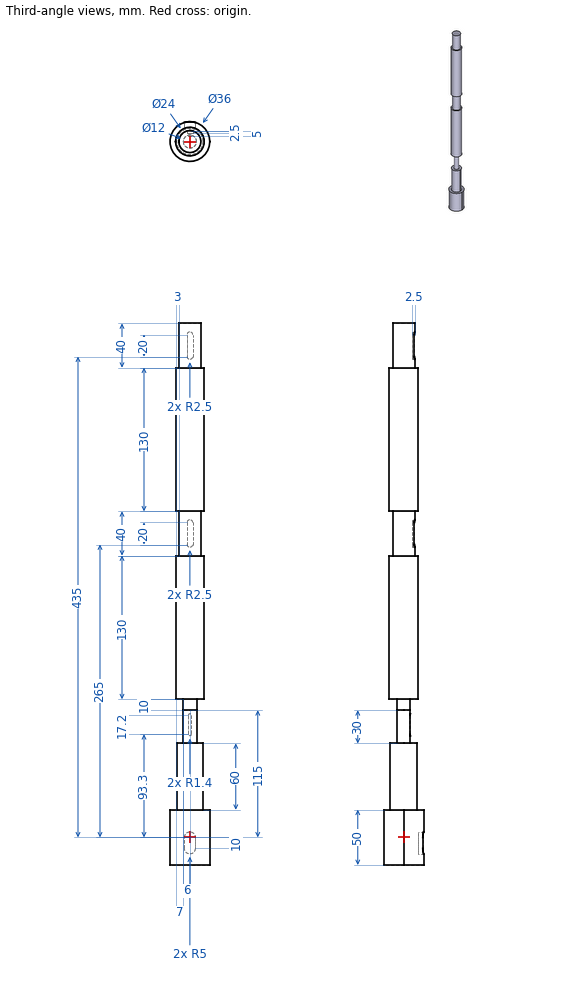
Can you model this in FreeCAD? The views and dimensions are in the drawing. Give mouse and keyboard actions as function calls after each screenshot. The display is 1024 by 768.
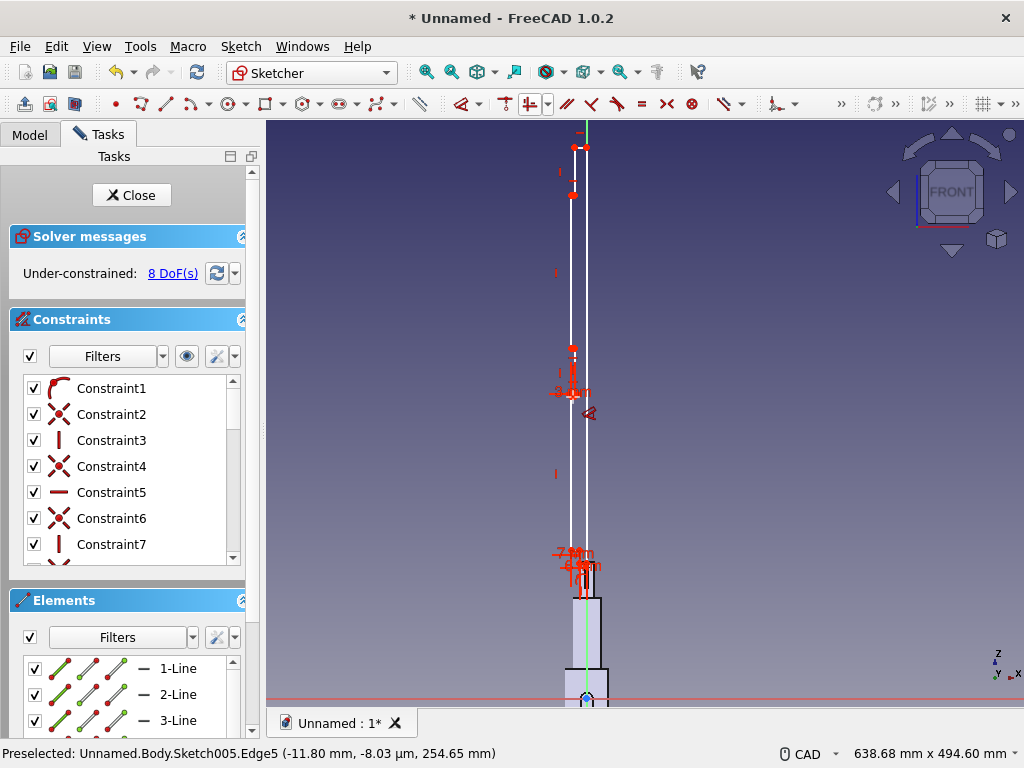
scroll(574, 365, up, 15)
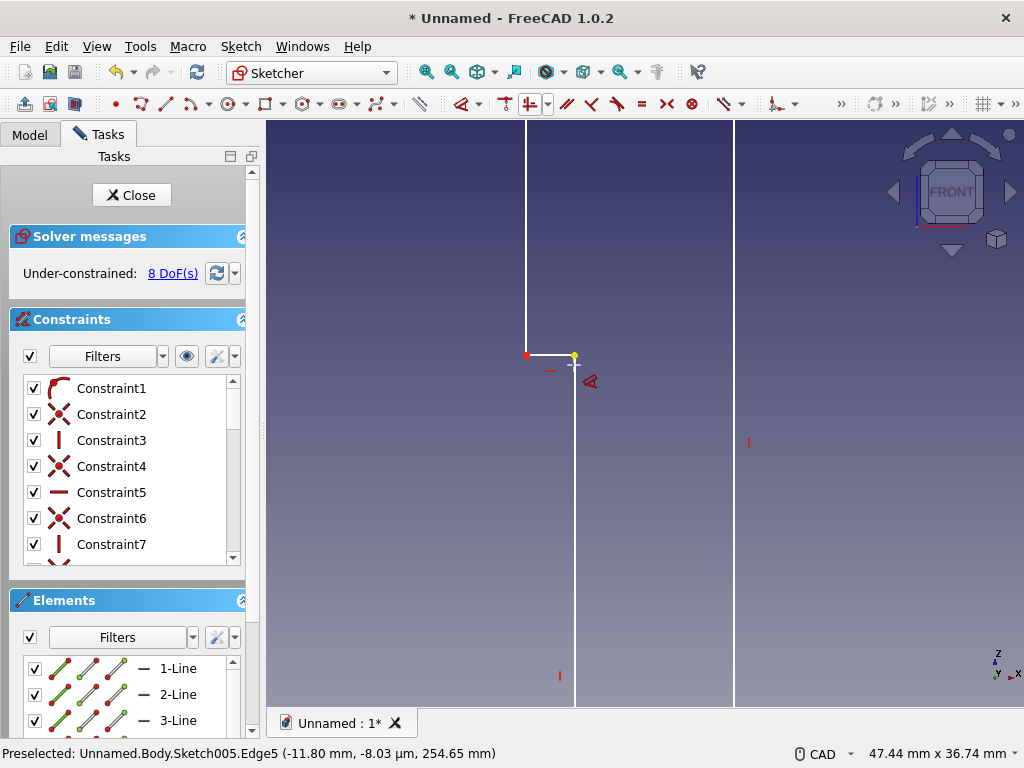
click(560, 355)
click(550, 321)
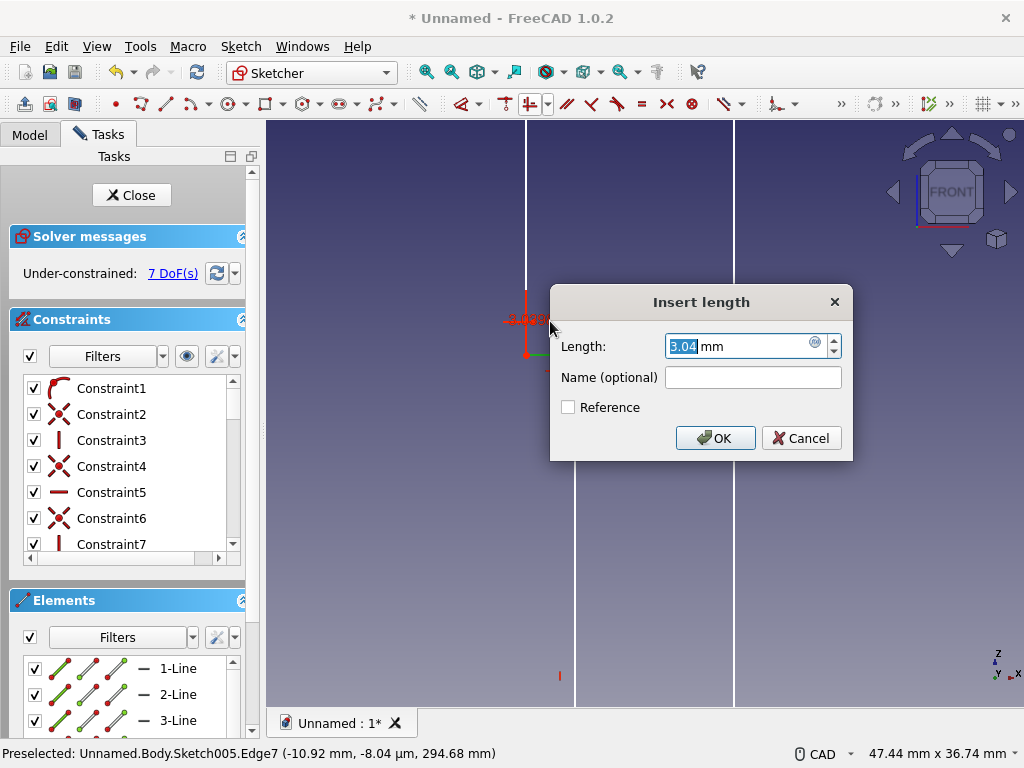
text(3)
key(Return)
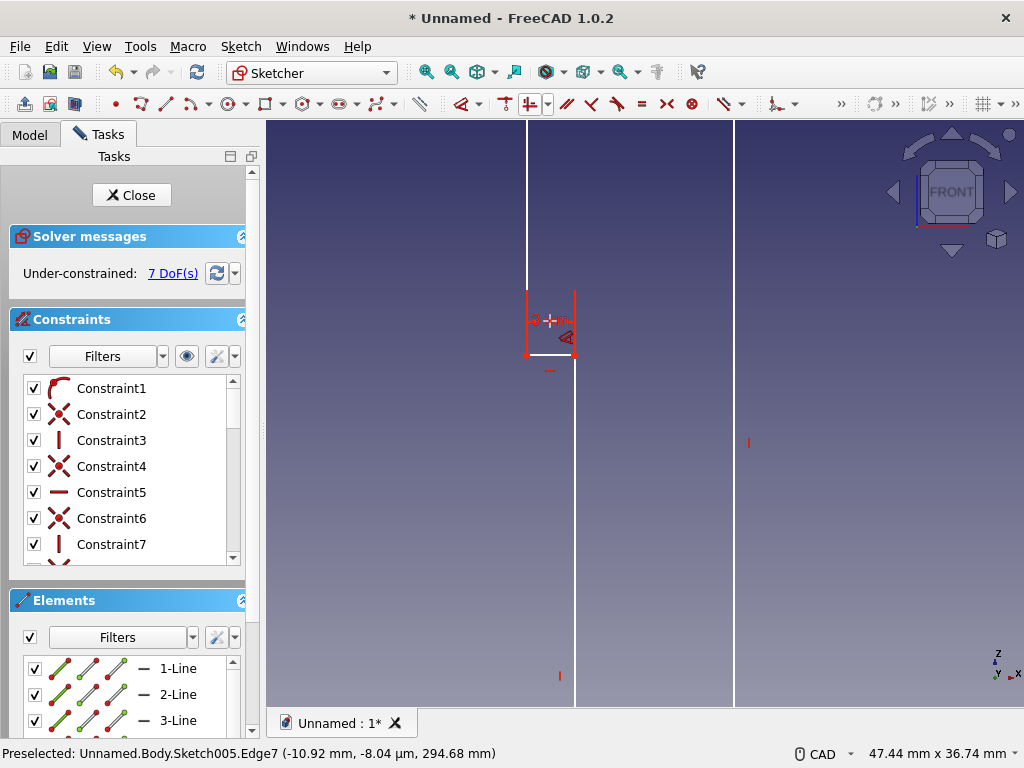
scroll(574, 364, down, 15)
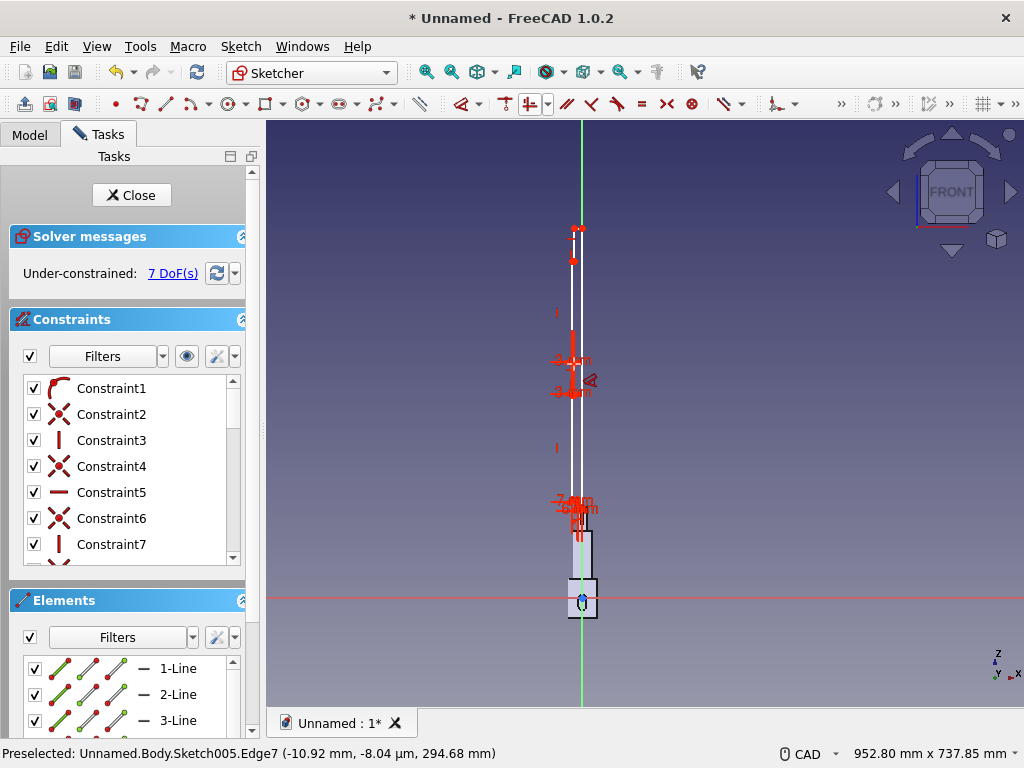
scroll(573, 261, up, 15)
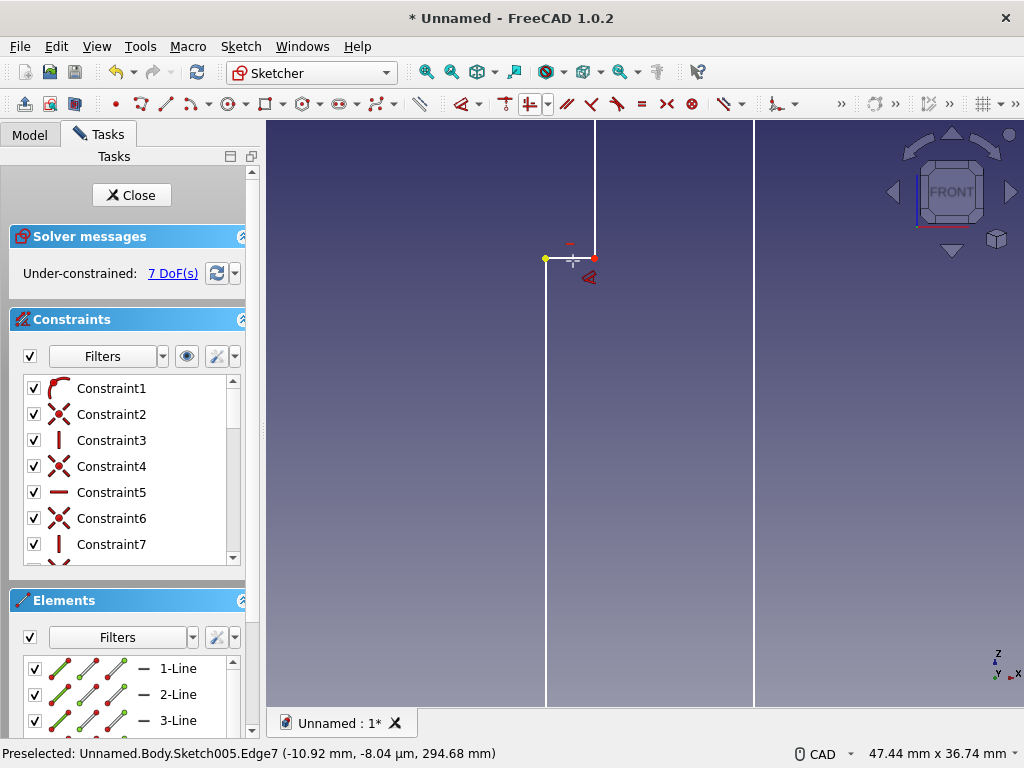
click(561, 258)
click(570, 224)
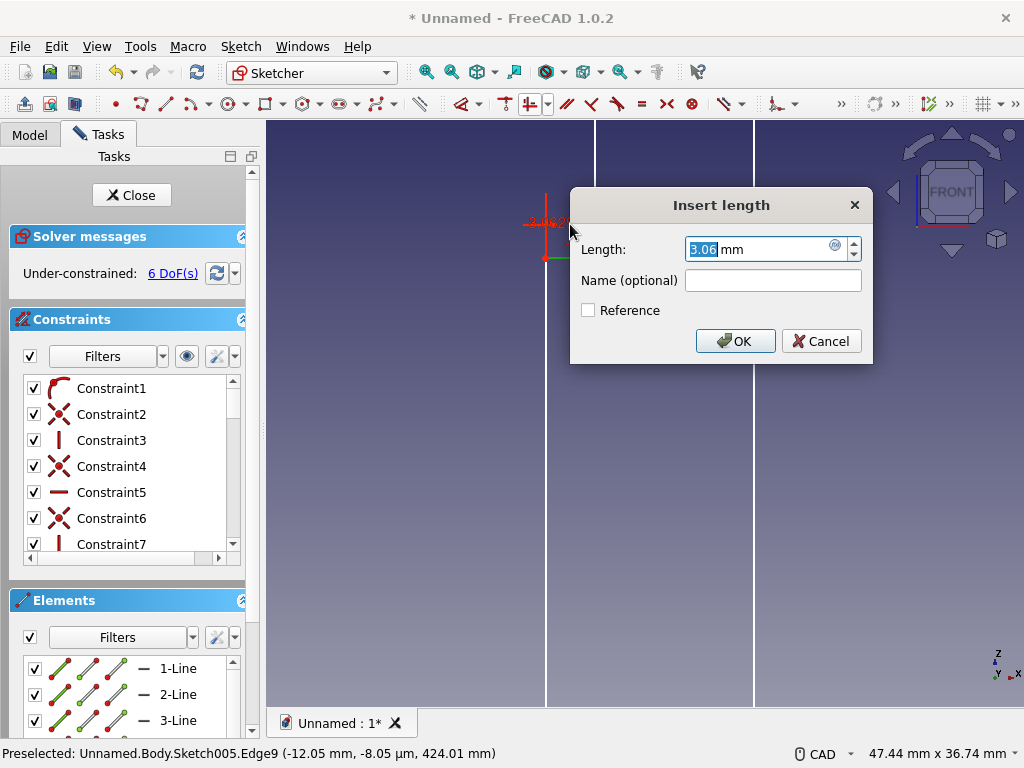
text(3)
key(Return)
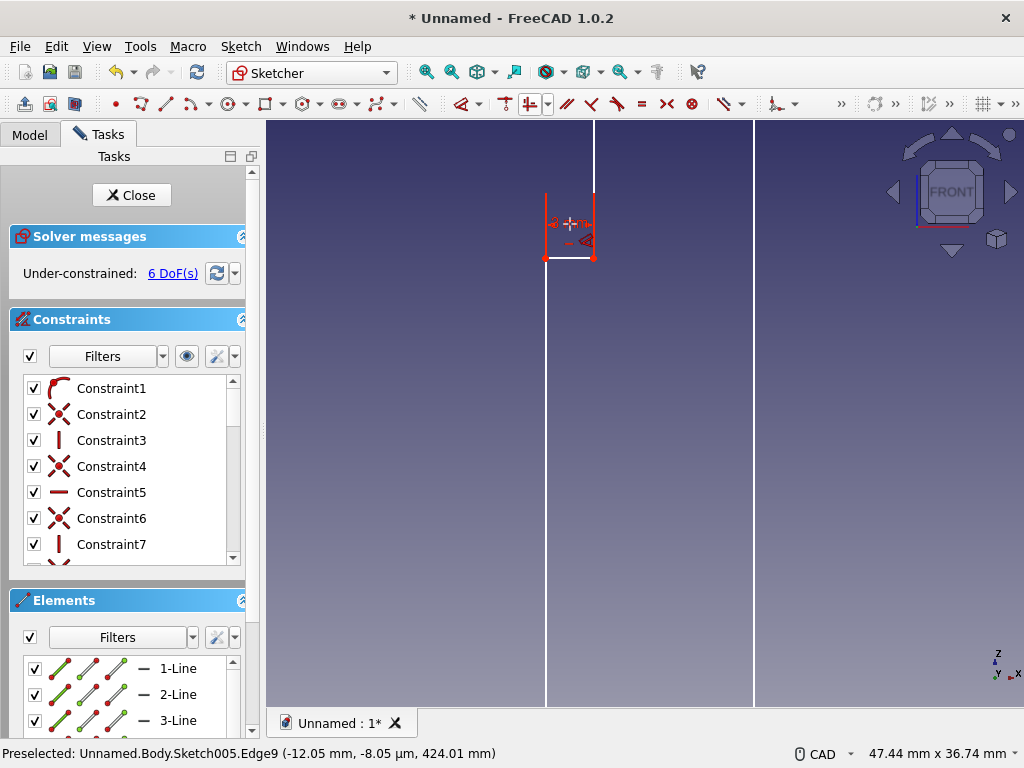
scroll(573, 261, down, 15)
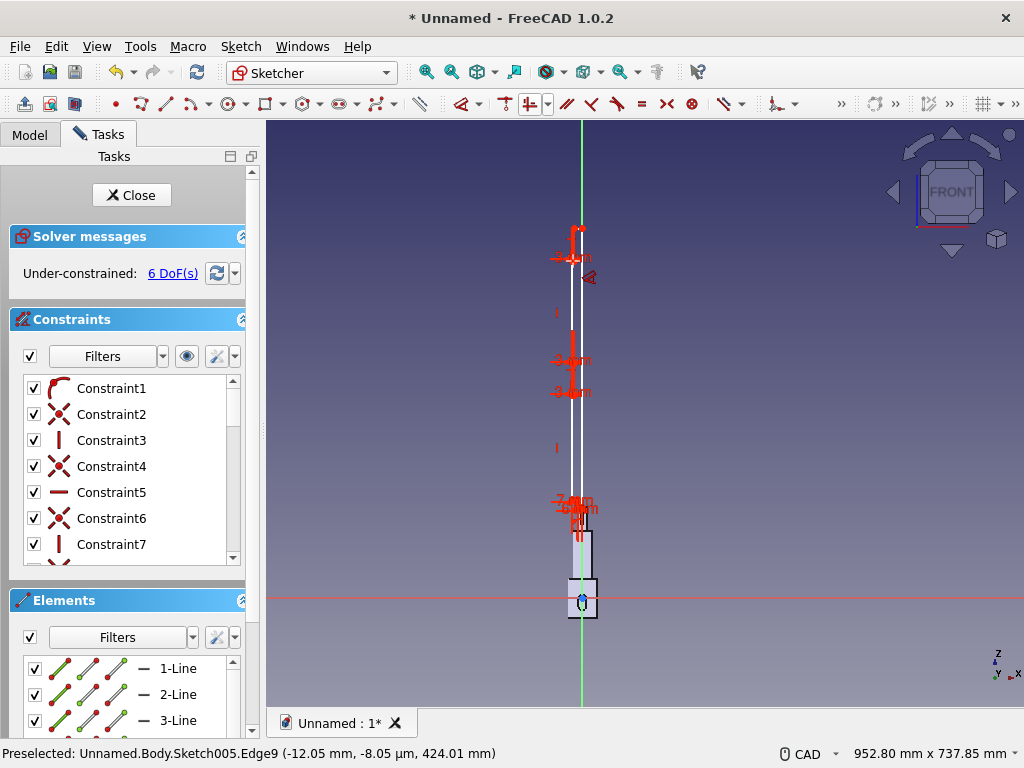
scroll(578, 505, up, 9)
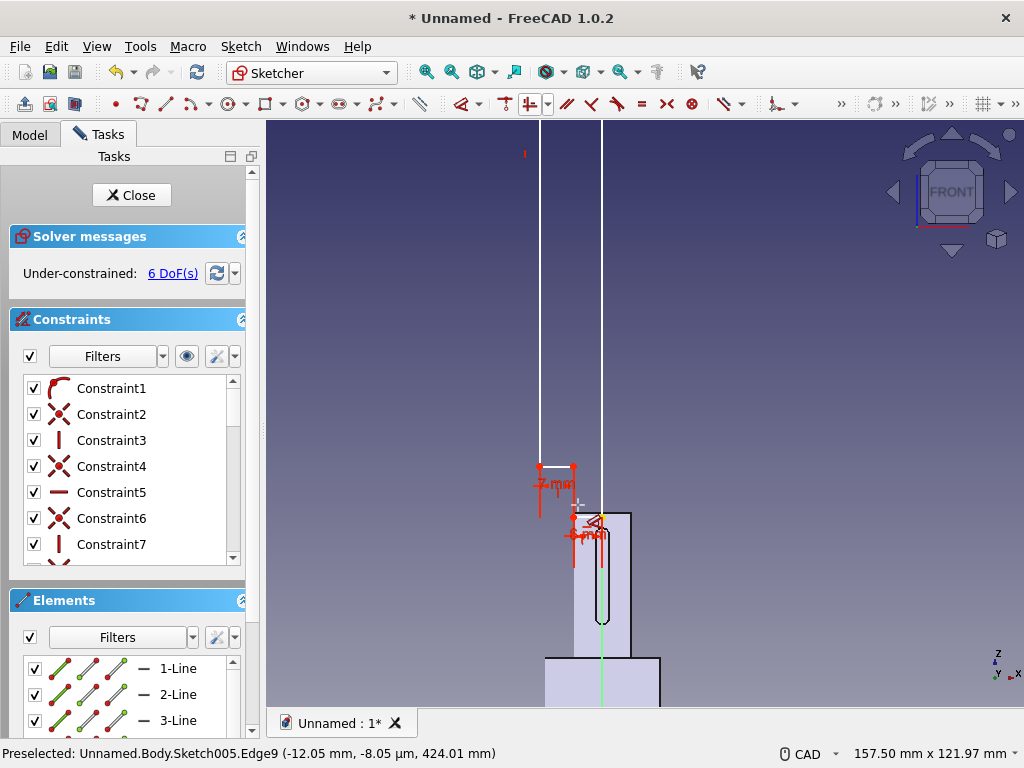
click(574, 502)
click(540, 510)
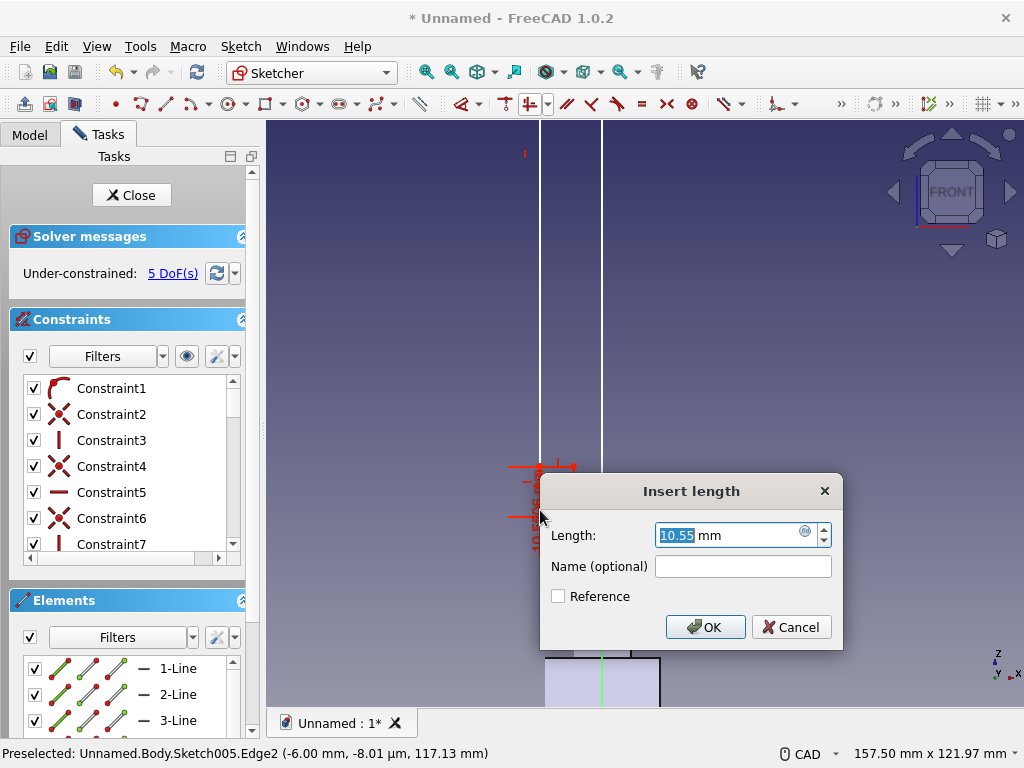
text(10)
key(Return)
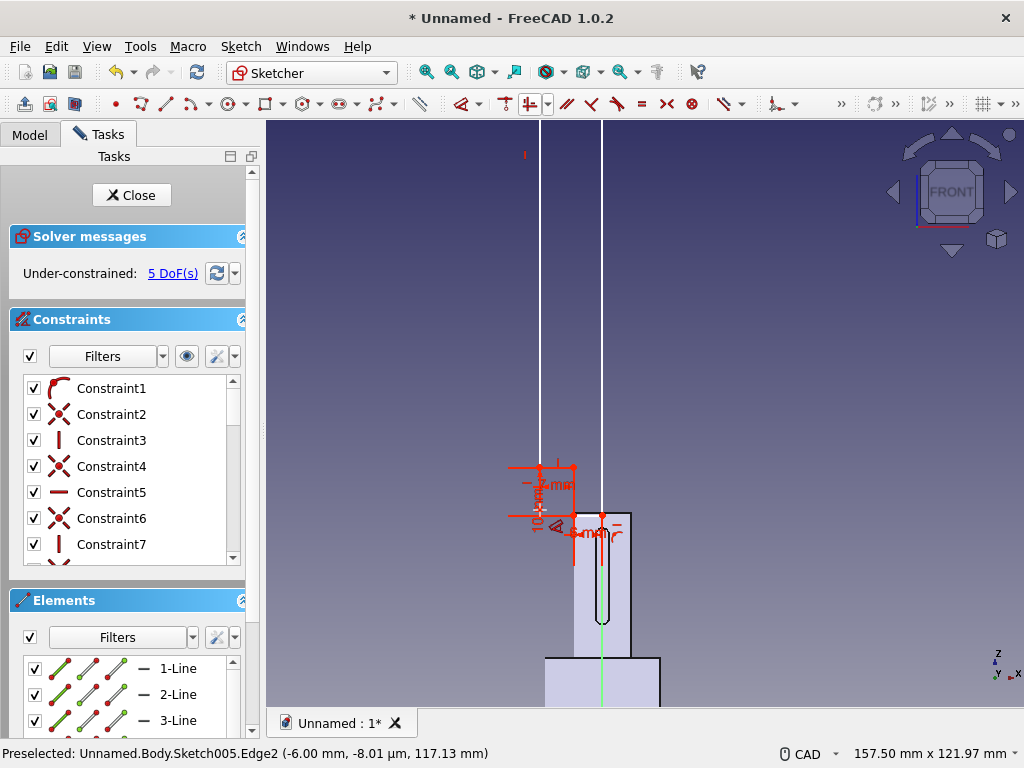
scroll(578, 506, down, 9)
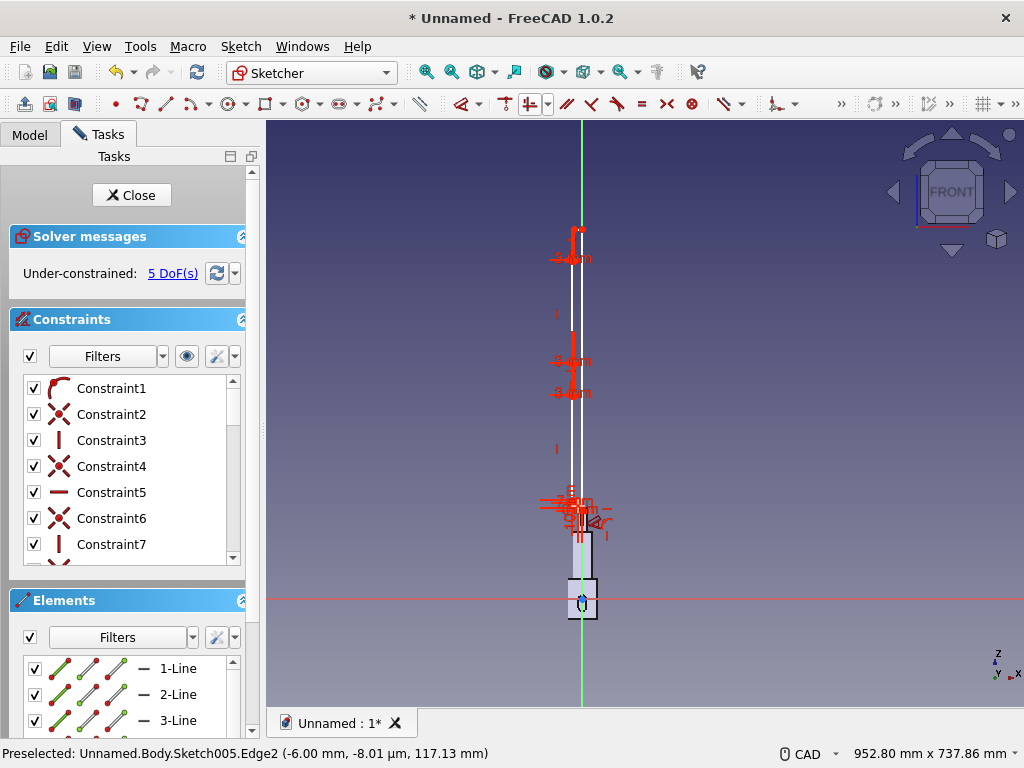
scroll(574, 387, up, 3)